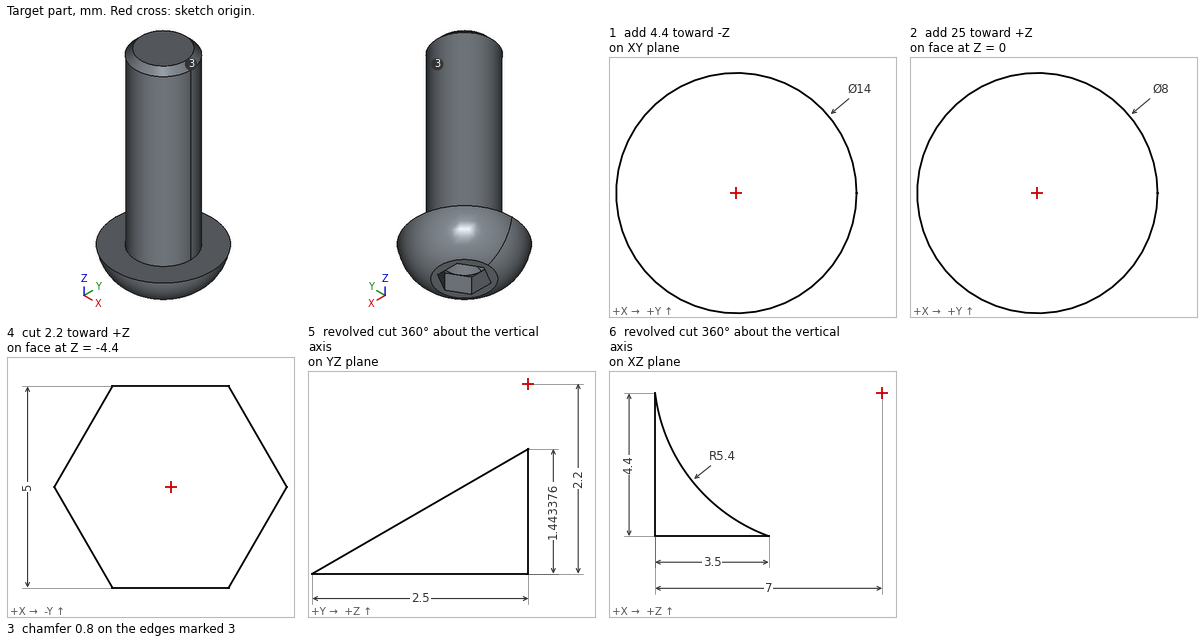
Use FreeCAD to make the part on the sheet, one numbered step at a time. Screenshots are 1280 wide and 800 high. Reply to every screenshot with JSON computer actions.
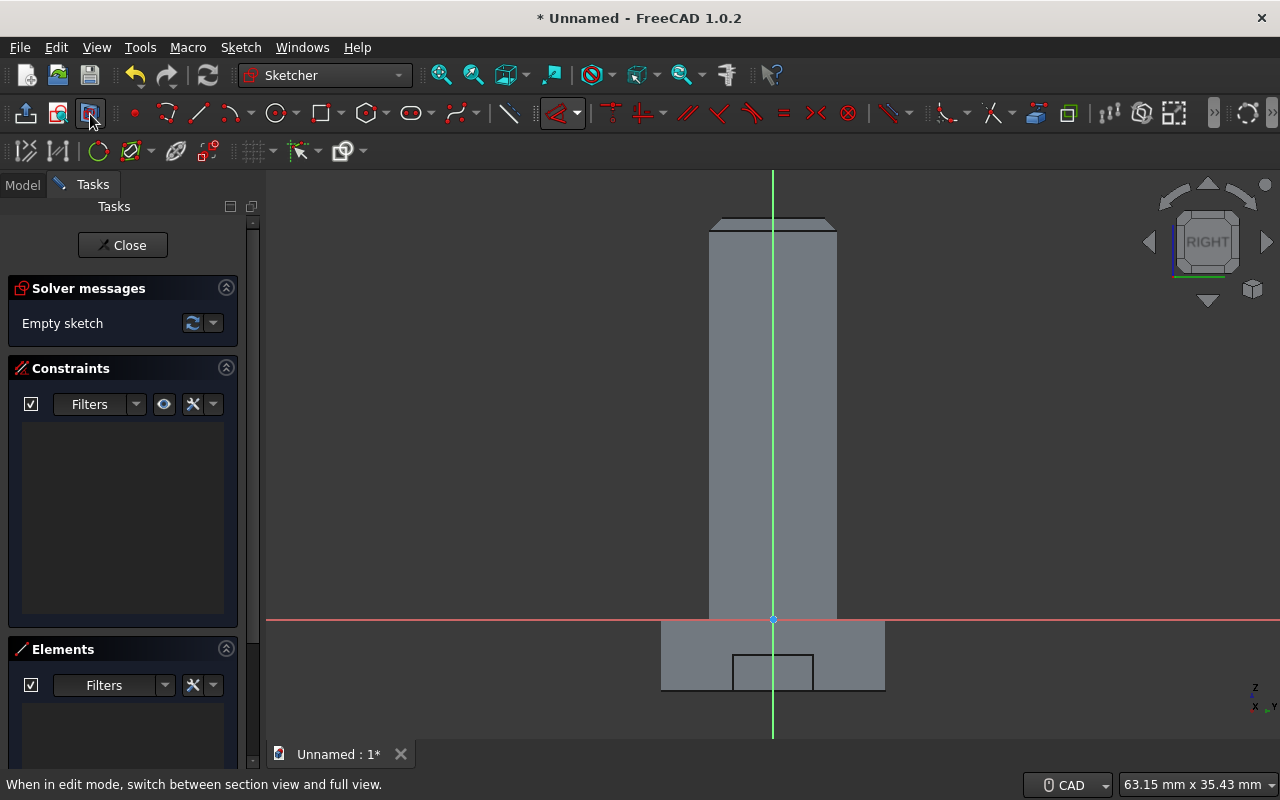
{"action": "scroll", "coordinate": [758, 656], "scroll_direction": "up", "scroll_amount": 12}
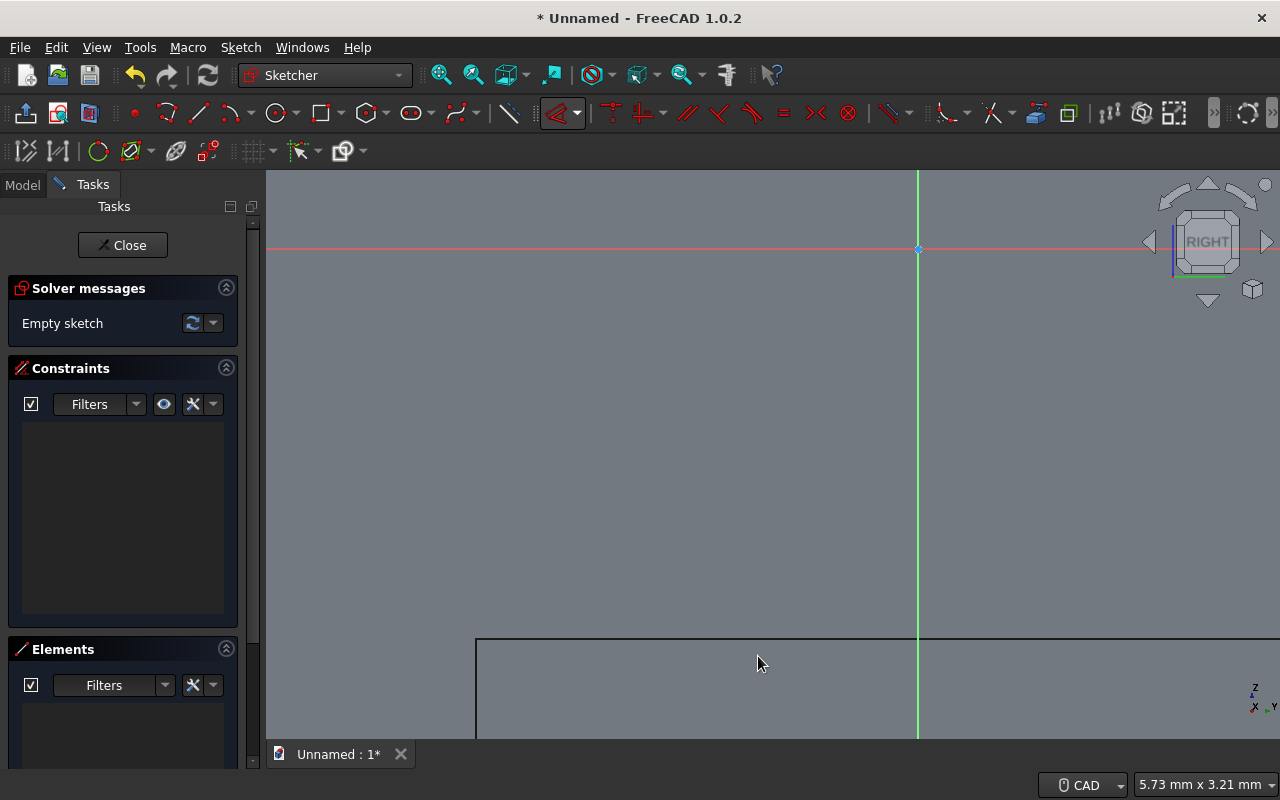
{"action": "key", "text": "g m"}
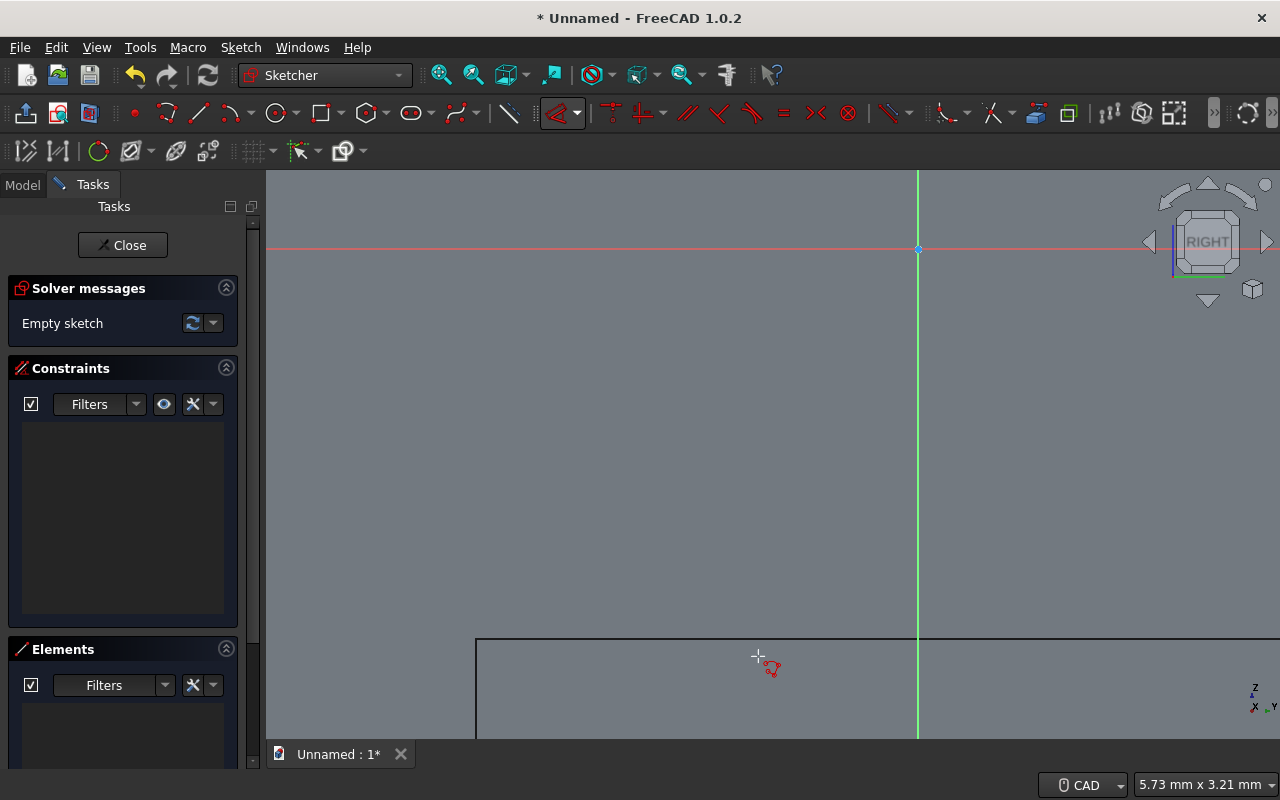
{"action": "left_click", "coordinate": [918, 383]}
{"action": "left_click", "coordinate": [909, 639]}
{"action": "left_click", "coordinate": [476, 639]}
{"action": "left_click", "coordinate": [918, 384]}
{"action": "key", "text": "Escape"}
{"action": "key", "text": "Escape"}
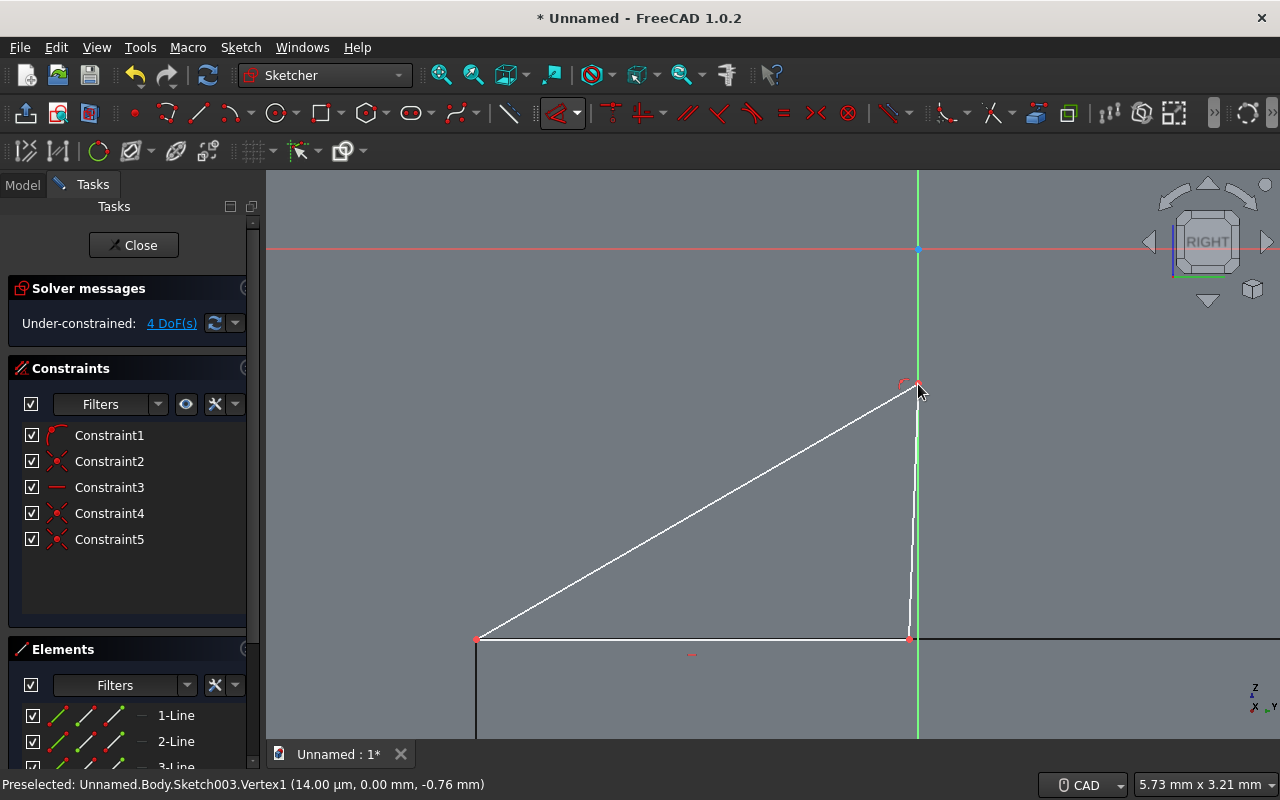
{"action": "left_click", "coordinate": [916, 461]}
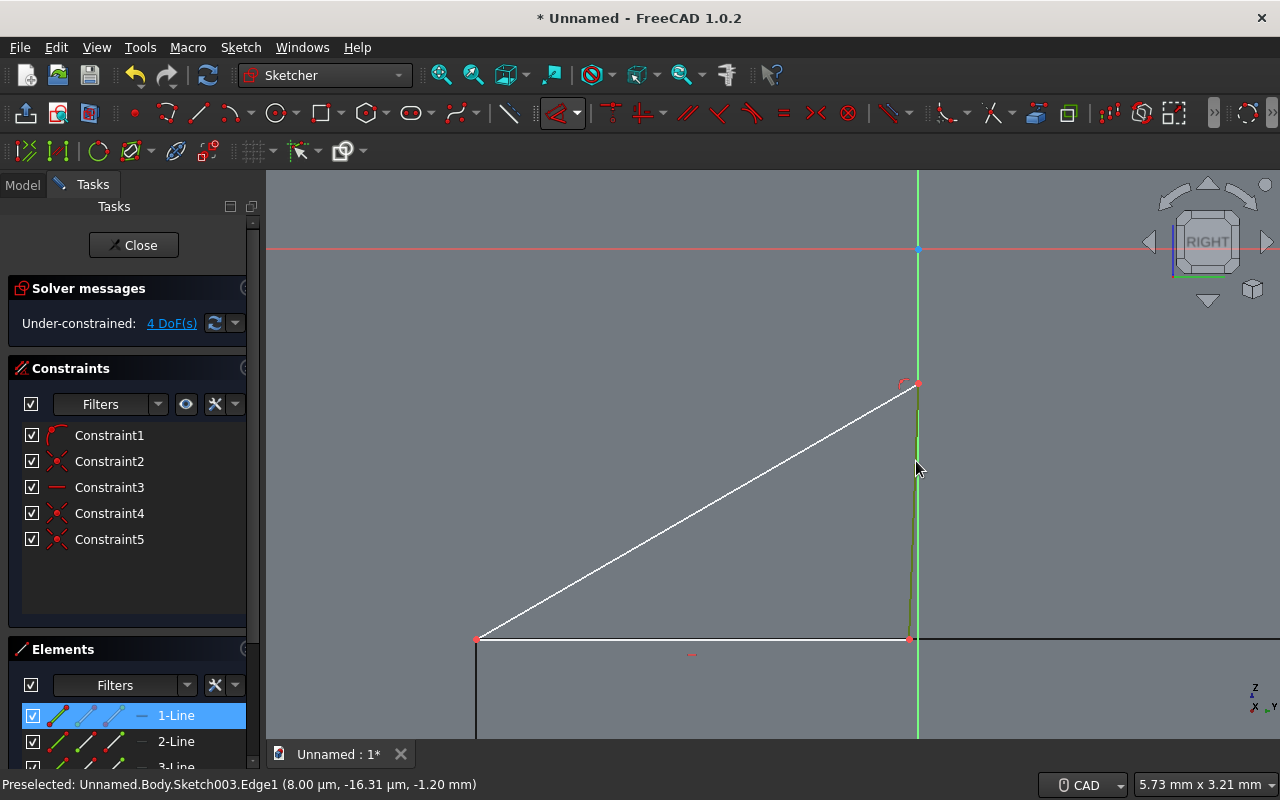
{"action": "left_click", "coordinate": [666, 114]}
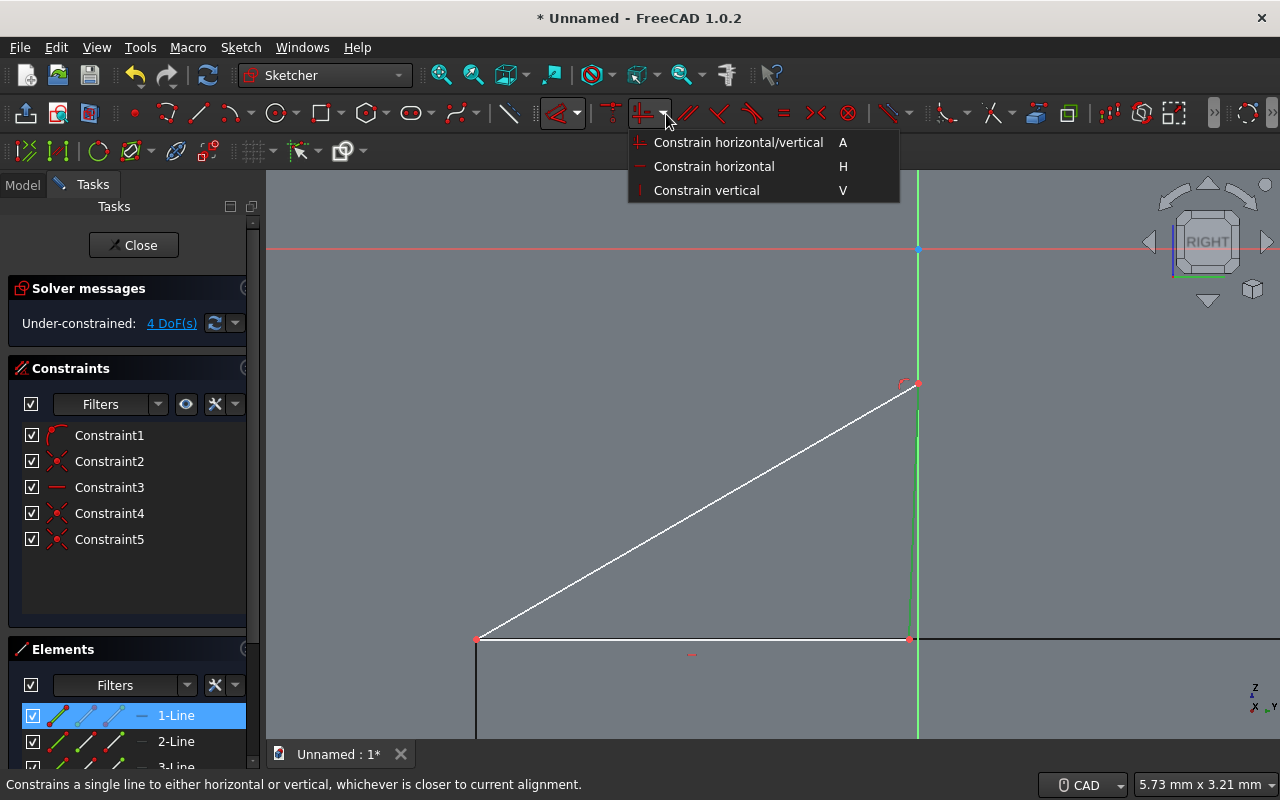
{"action": "left_click", "coordinate": [764, 190]}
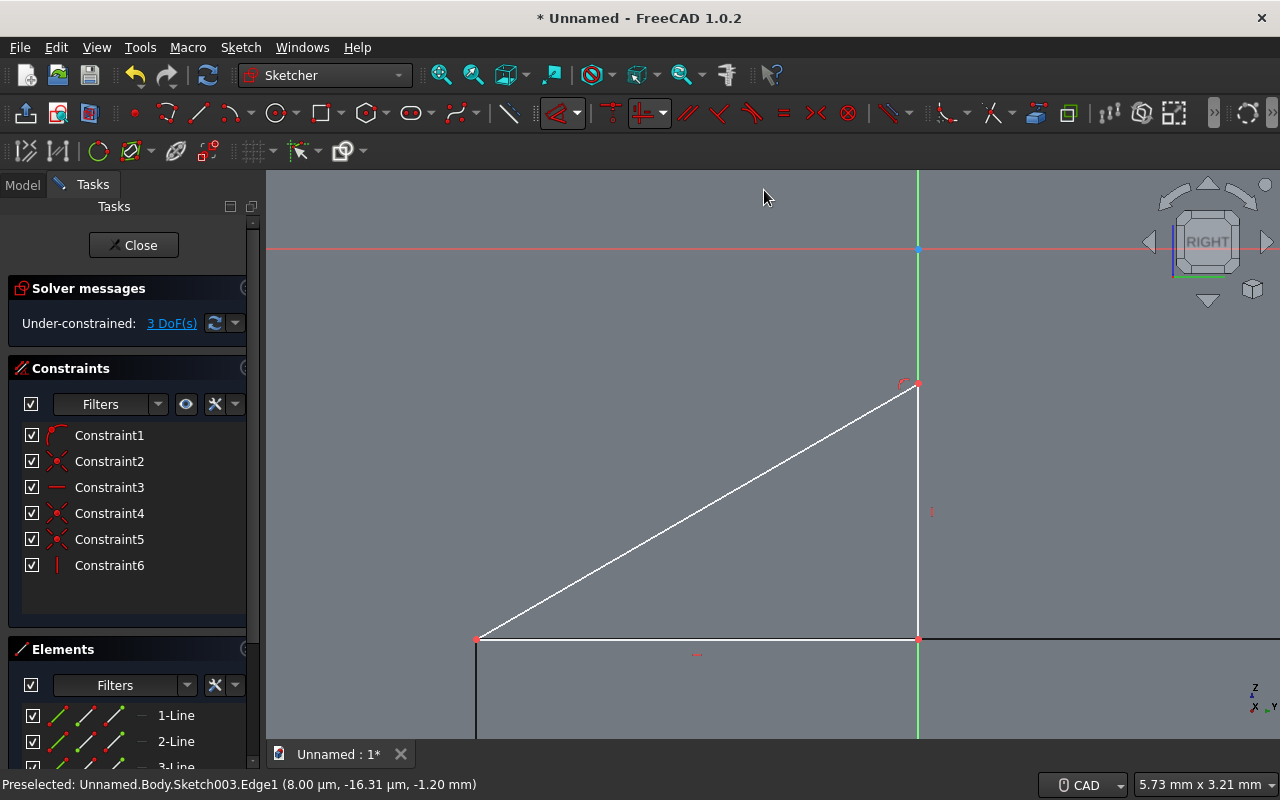
{"action": "left_click", "coordinate": [786, 640]}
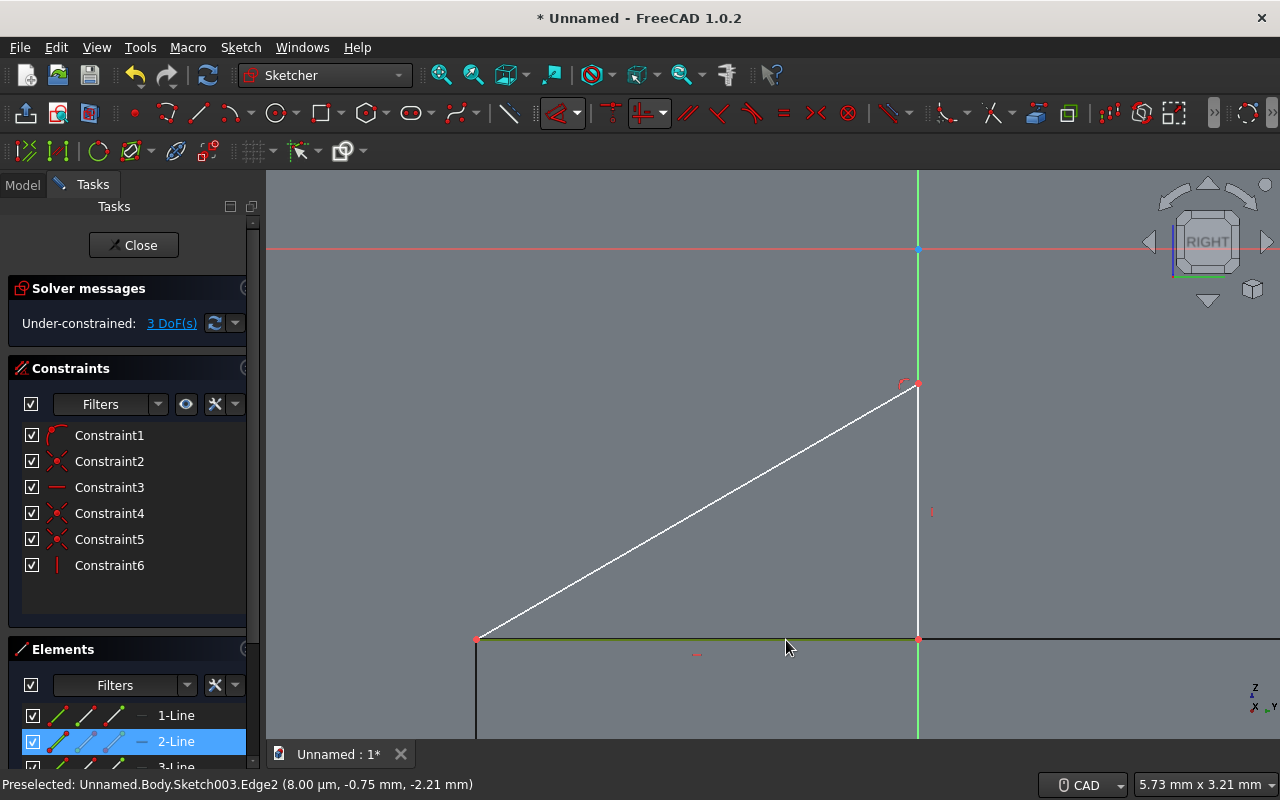
{"action": "left_click", "coordinate": [580, 114]}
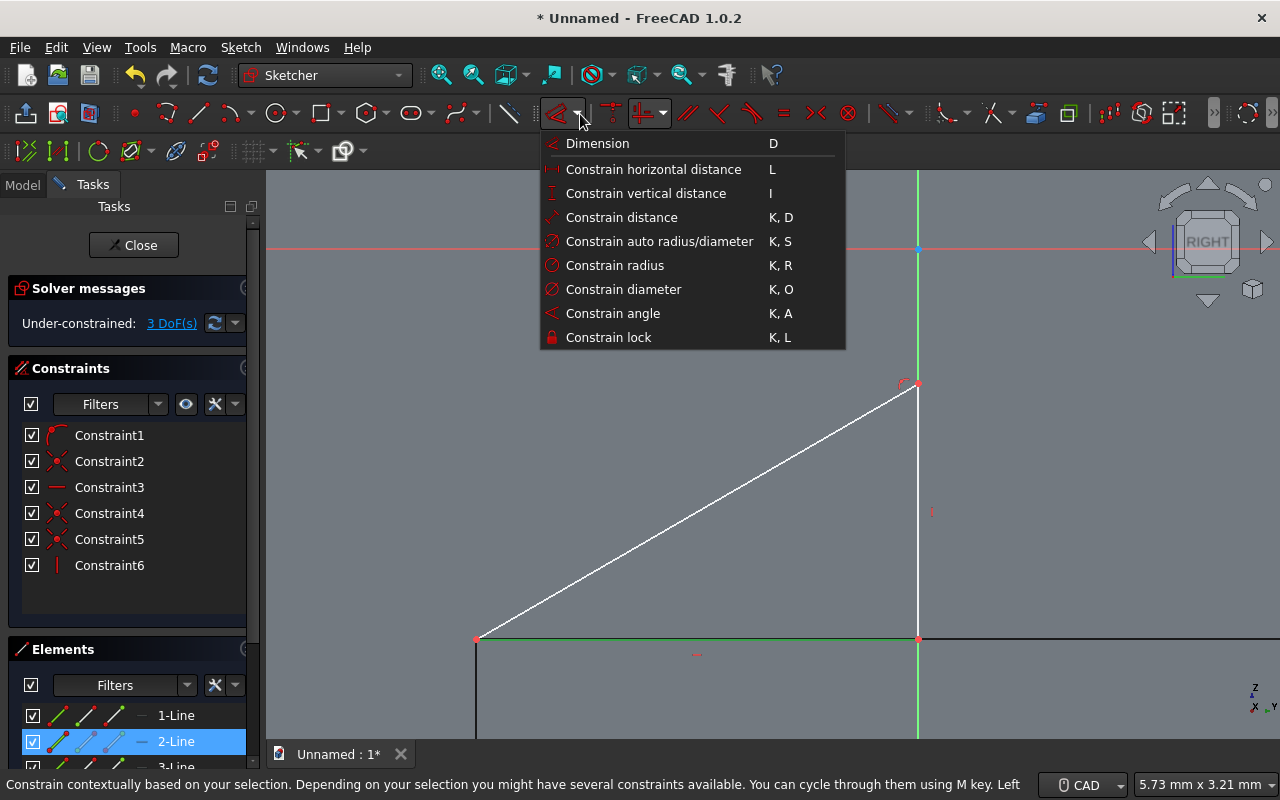
{"action": "left_click", "coordinate": [693, 169]}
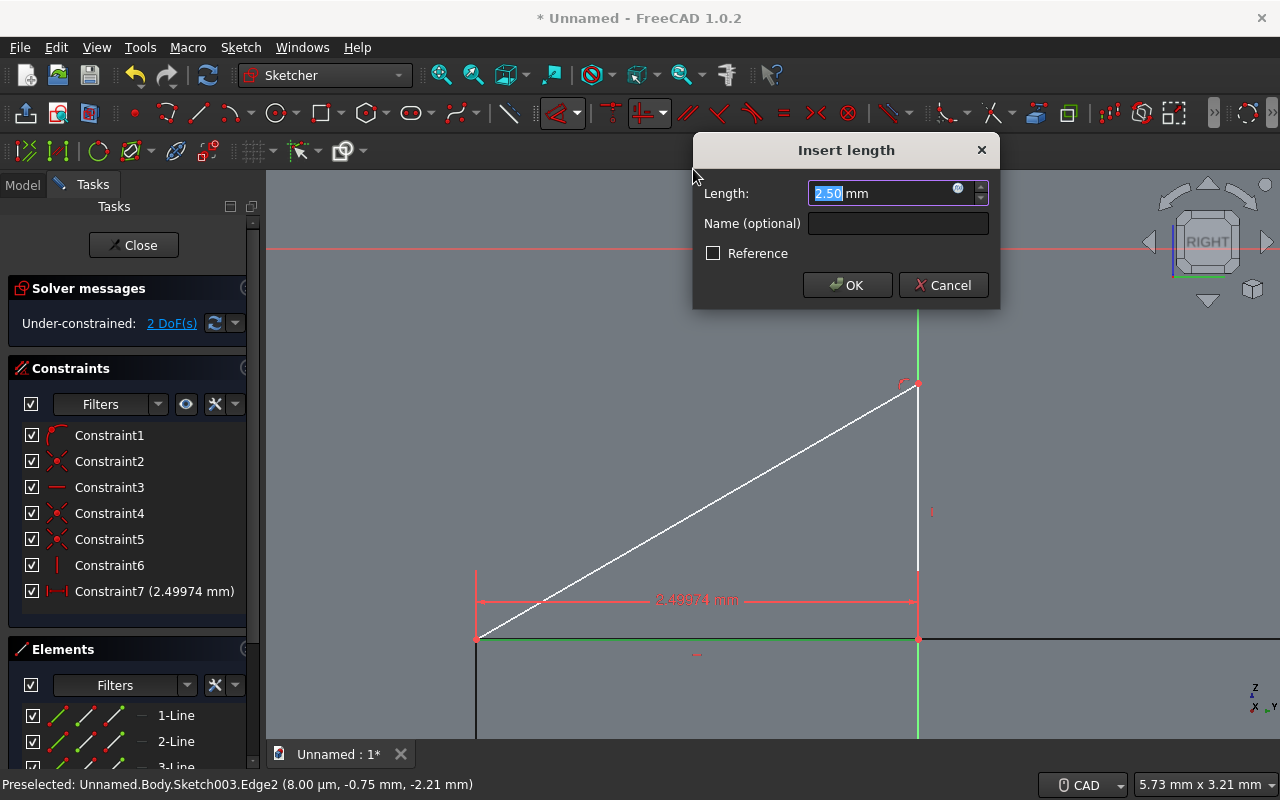
{"action": "type", "text": "2.5"}
{"action": "key", "text": "Return"}